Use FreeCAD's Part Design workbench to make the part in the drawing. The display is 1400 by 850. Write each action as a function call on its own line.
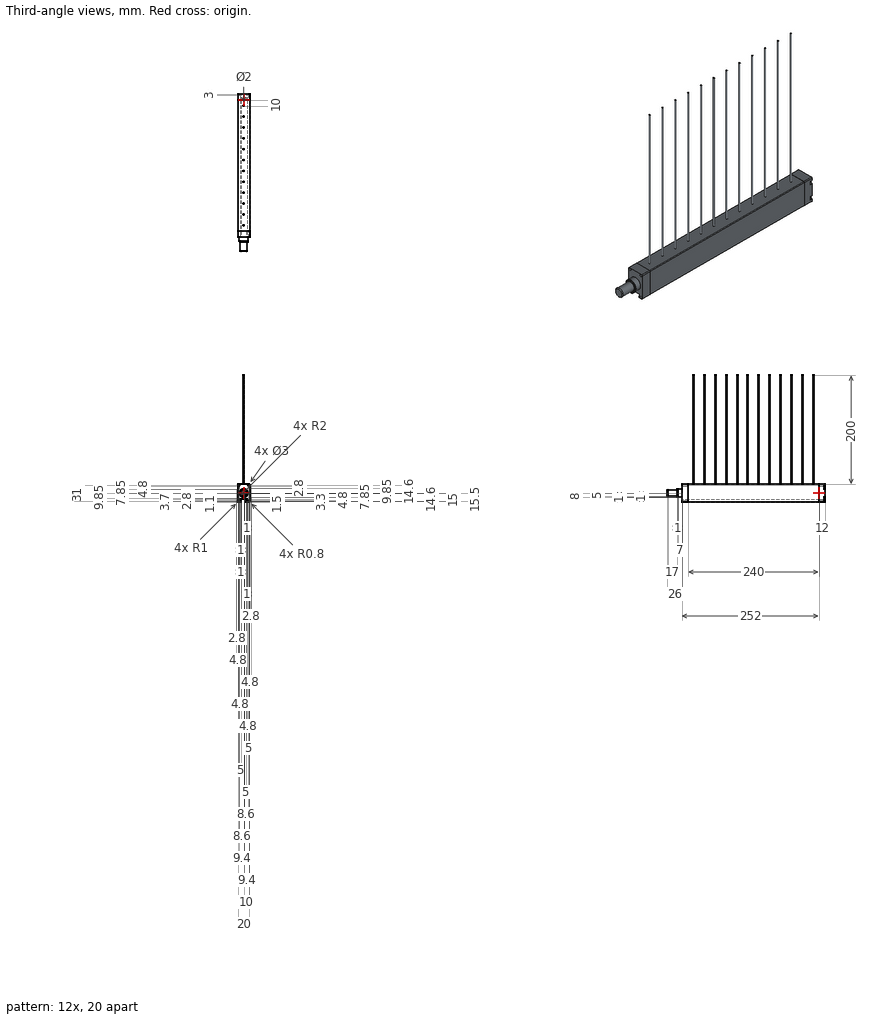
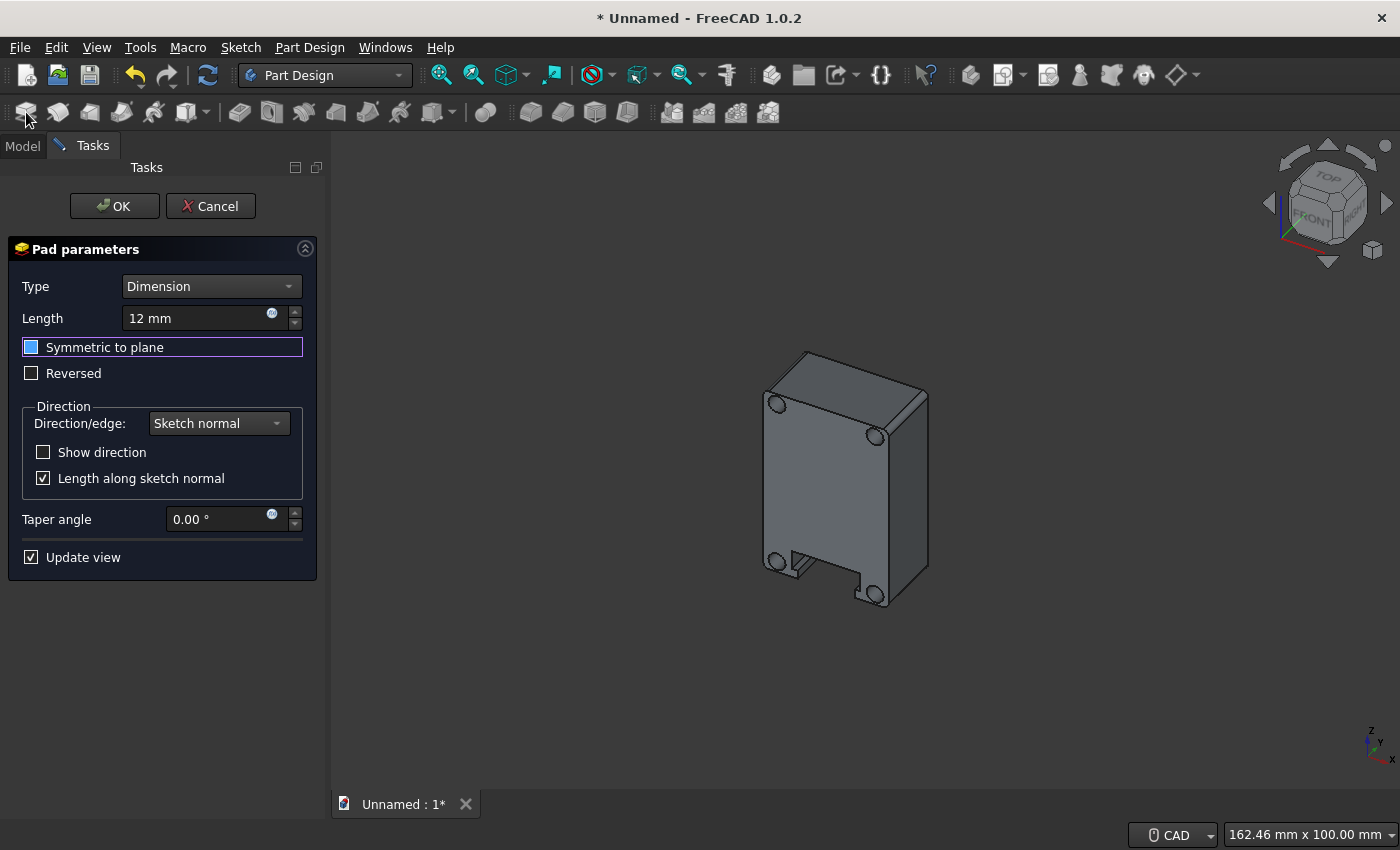
click(30, 373)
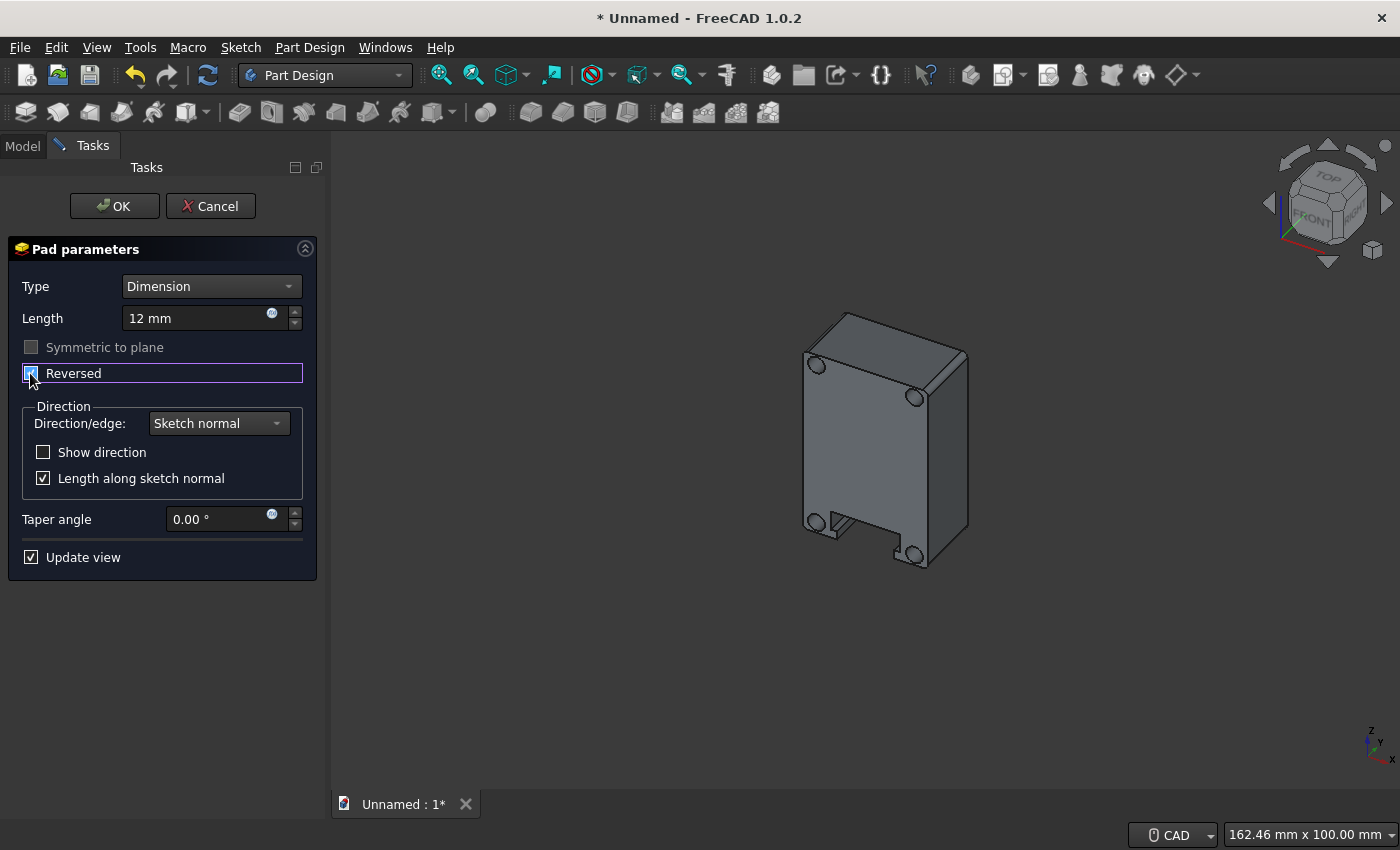
click(115, 206)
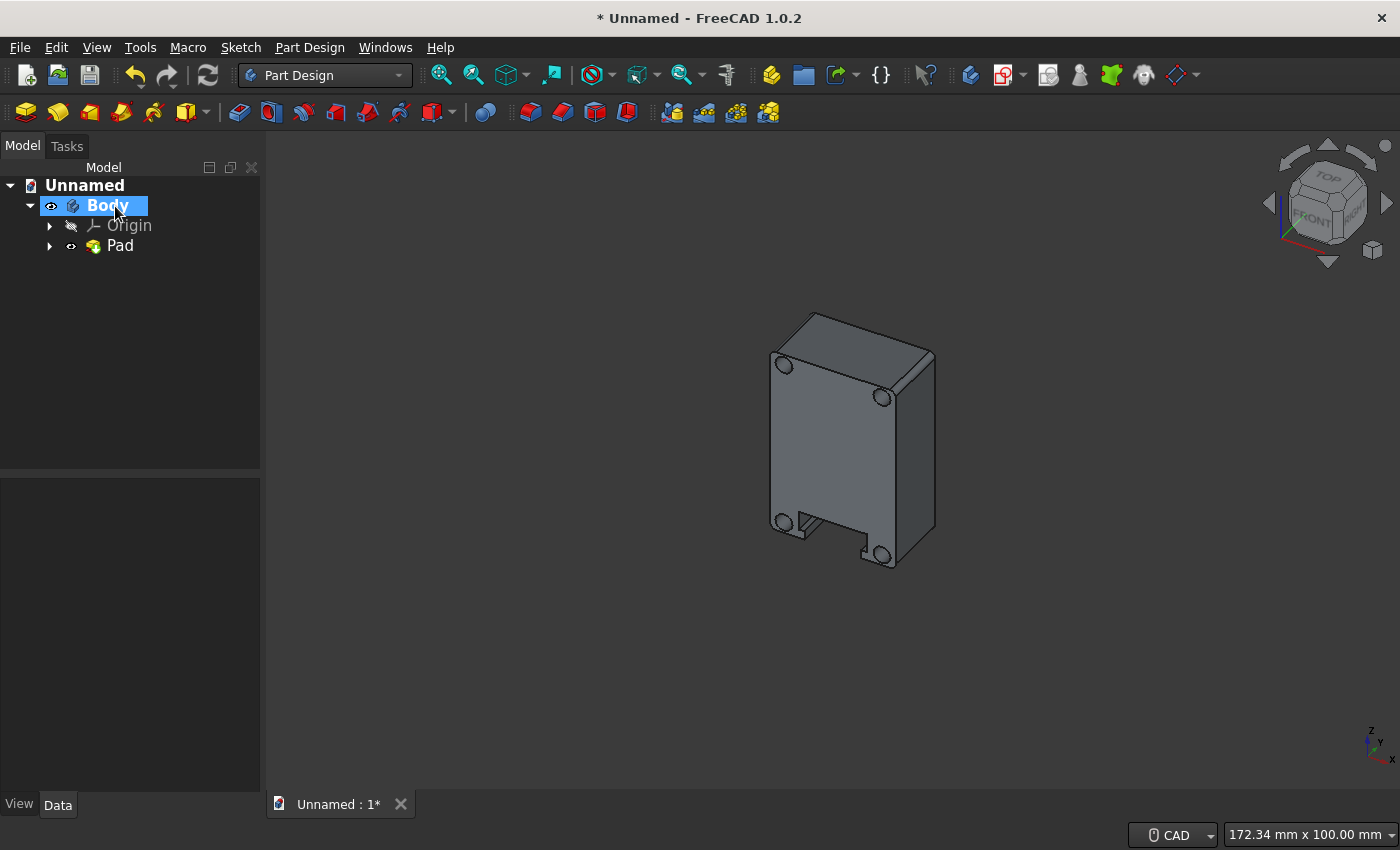
click(442, 76)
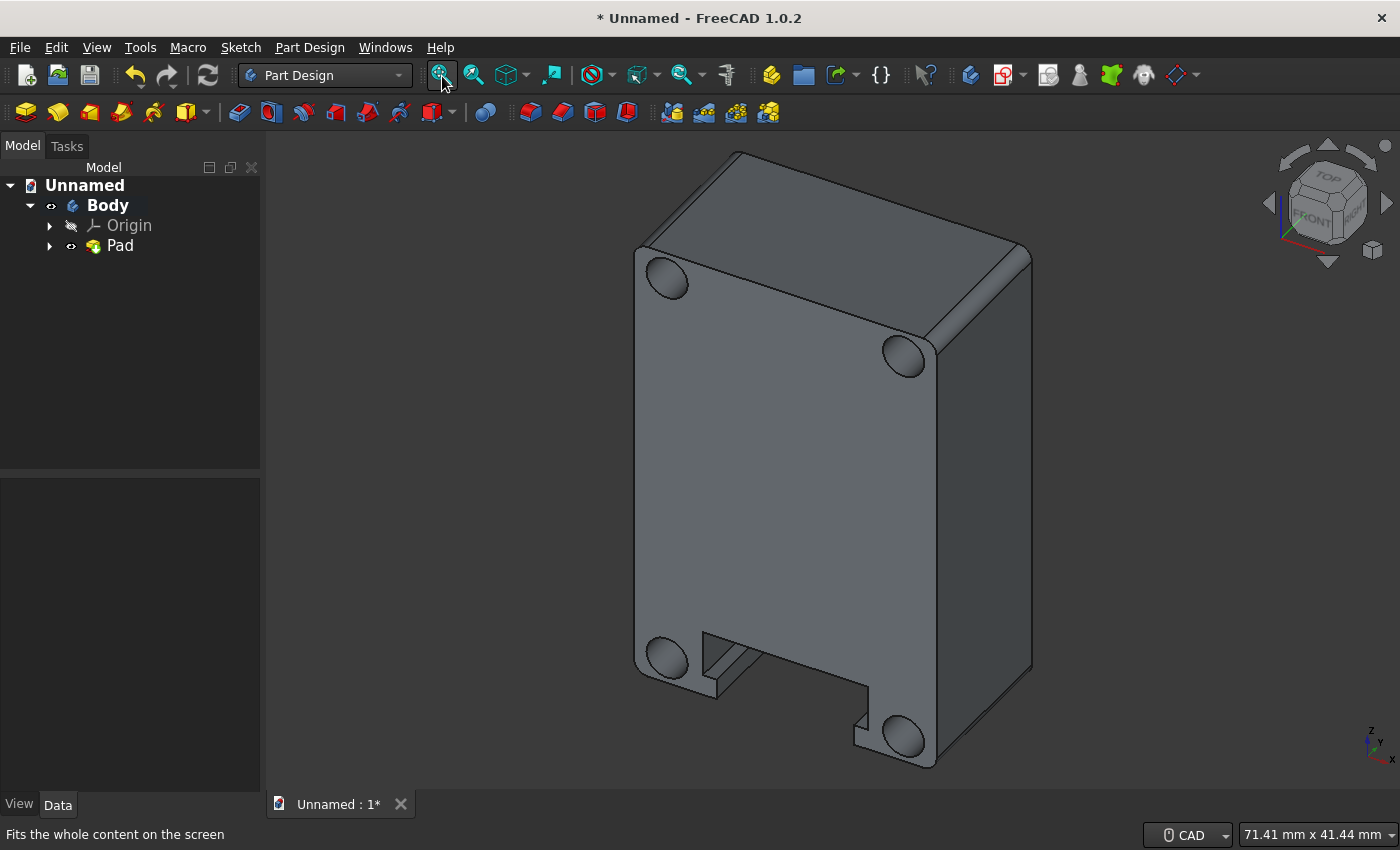
key(4)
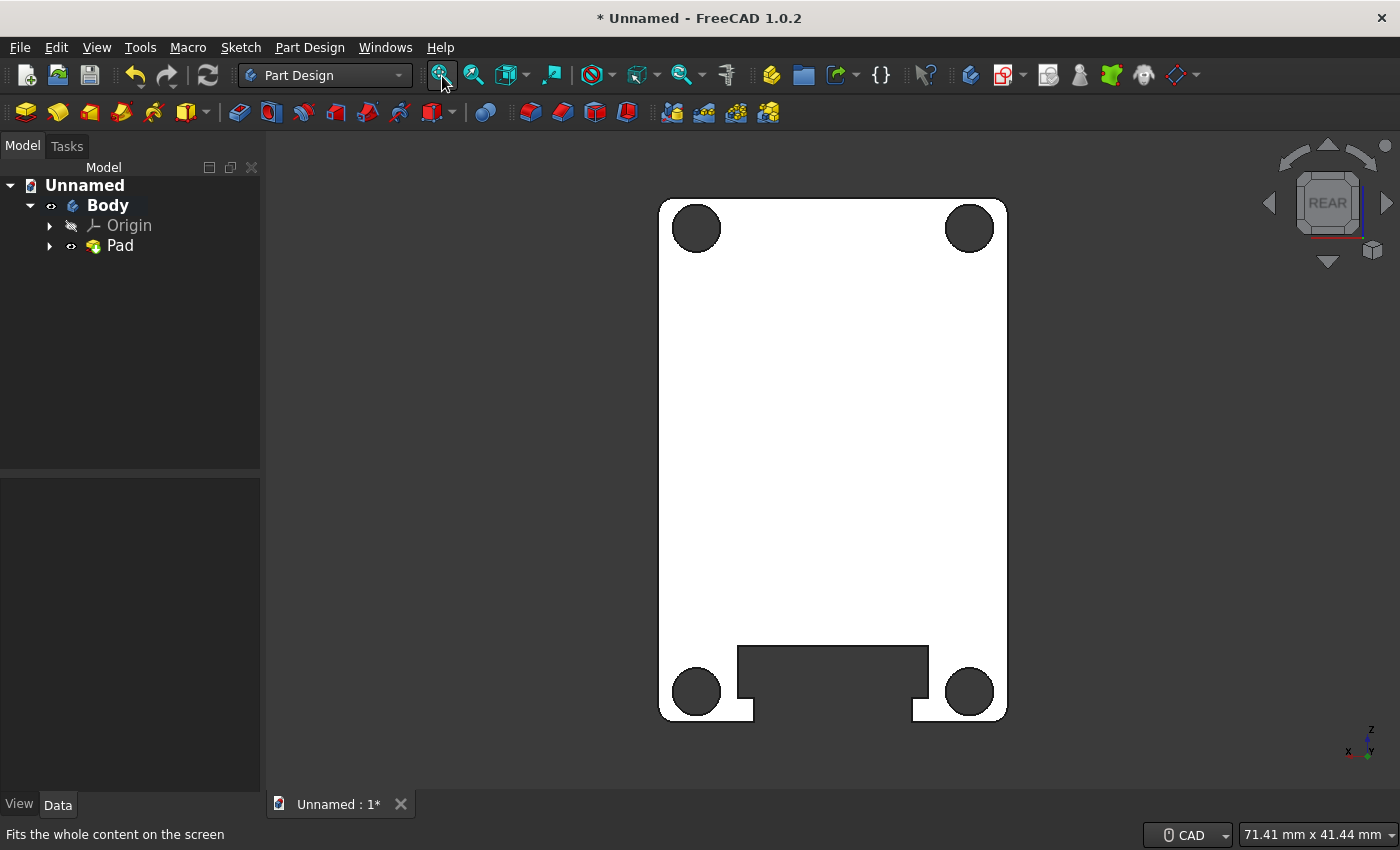
click(833, 384)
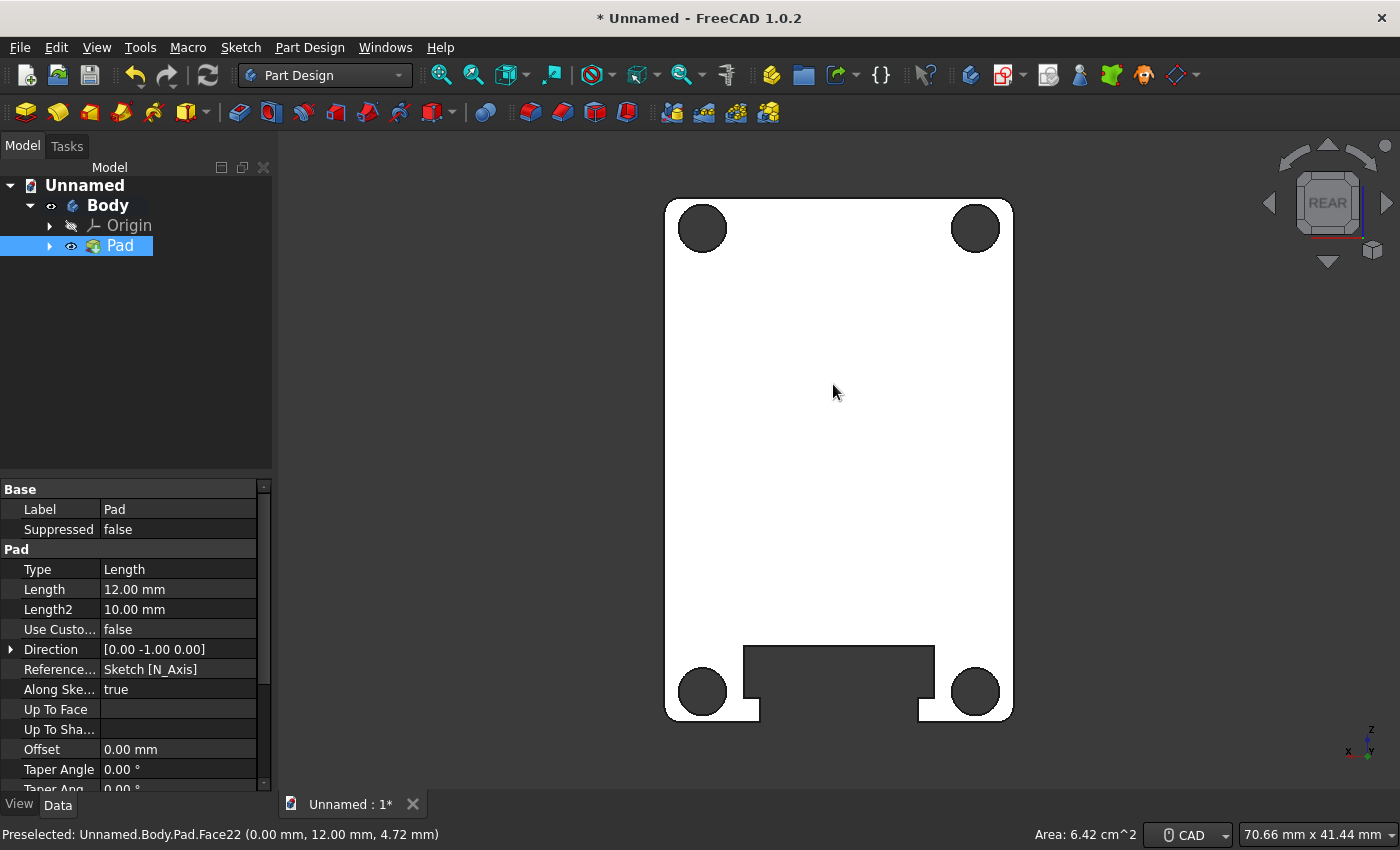
click(1004, 76)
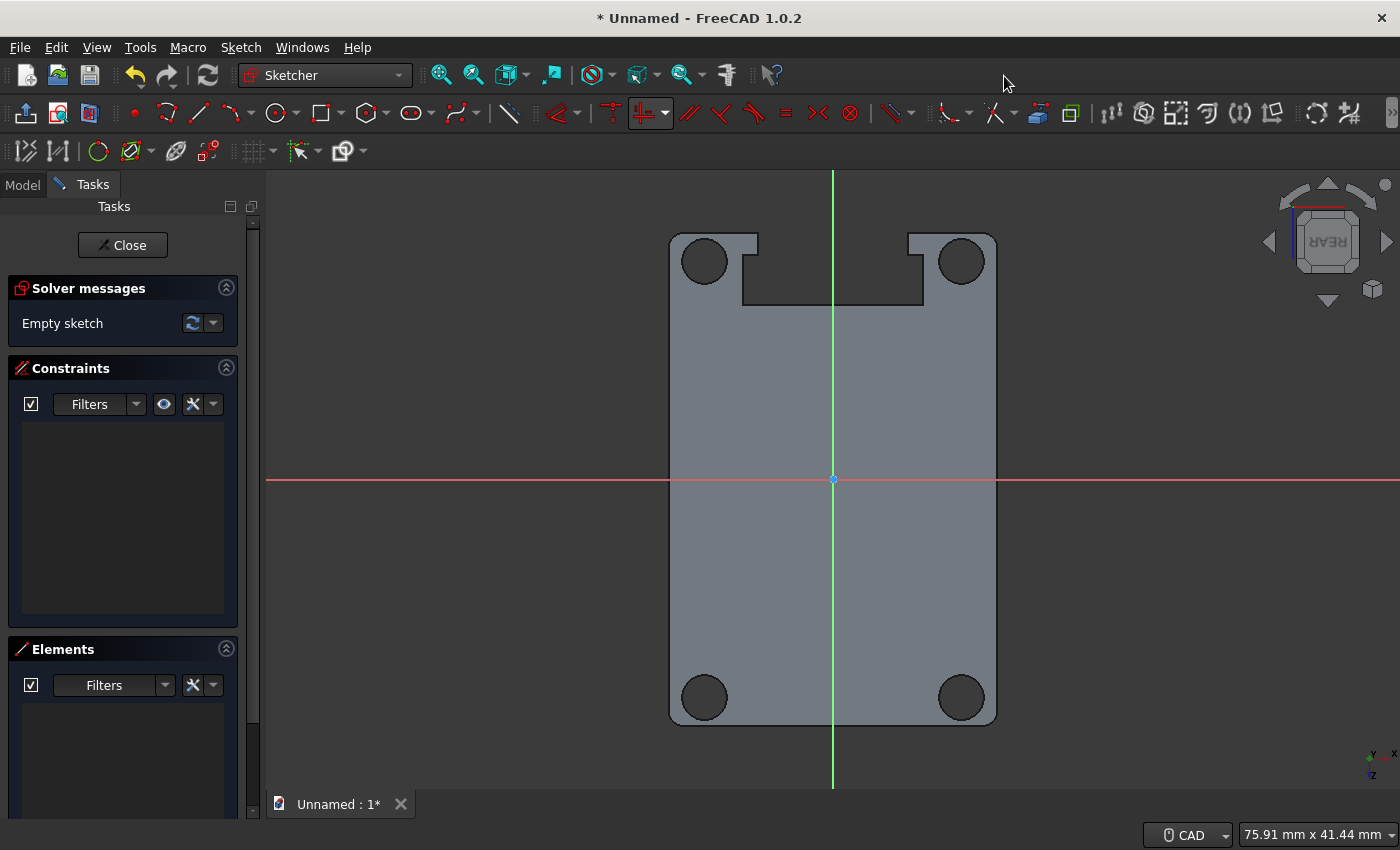
key(g)
key(m)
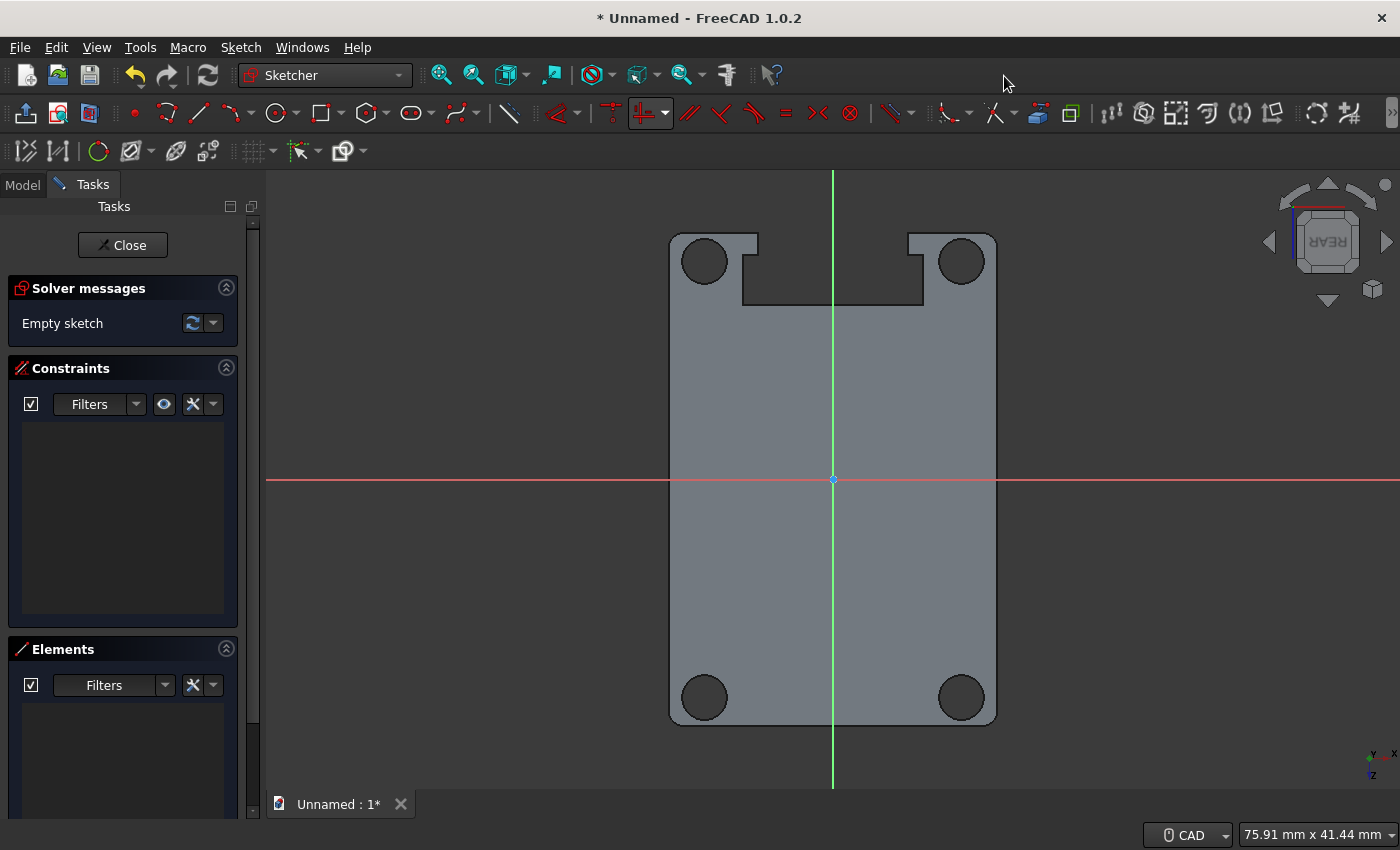
click(693, 332)
click(693, 291)
click(621, 291)
click(621, 362)
click(663, 362)
right_click(663, 362)